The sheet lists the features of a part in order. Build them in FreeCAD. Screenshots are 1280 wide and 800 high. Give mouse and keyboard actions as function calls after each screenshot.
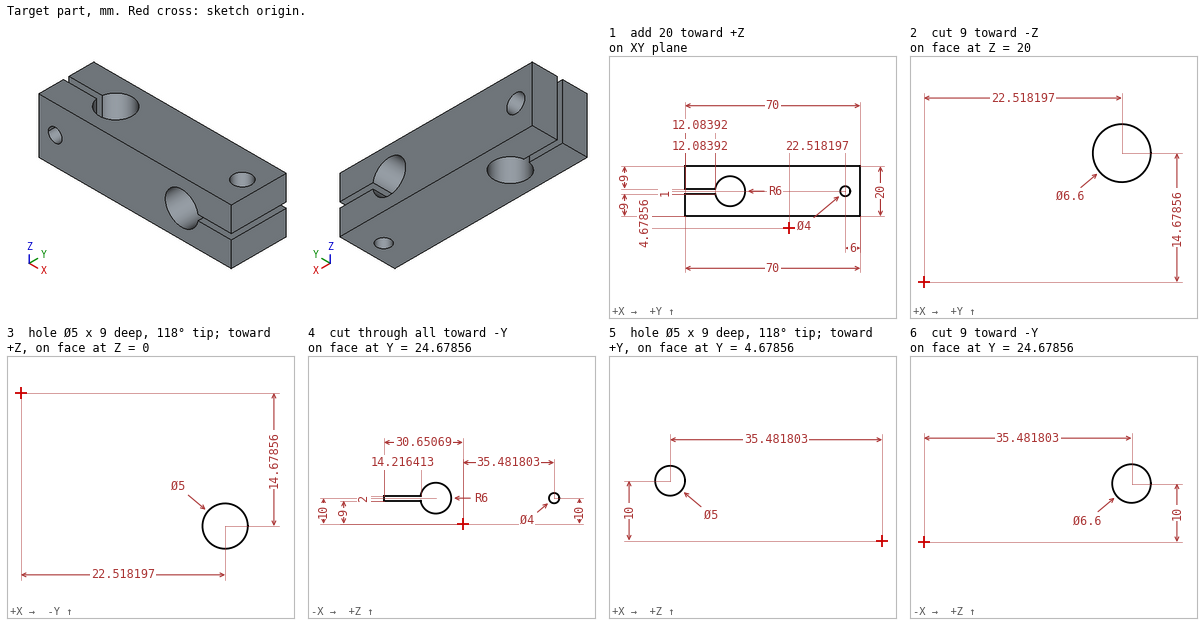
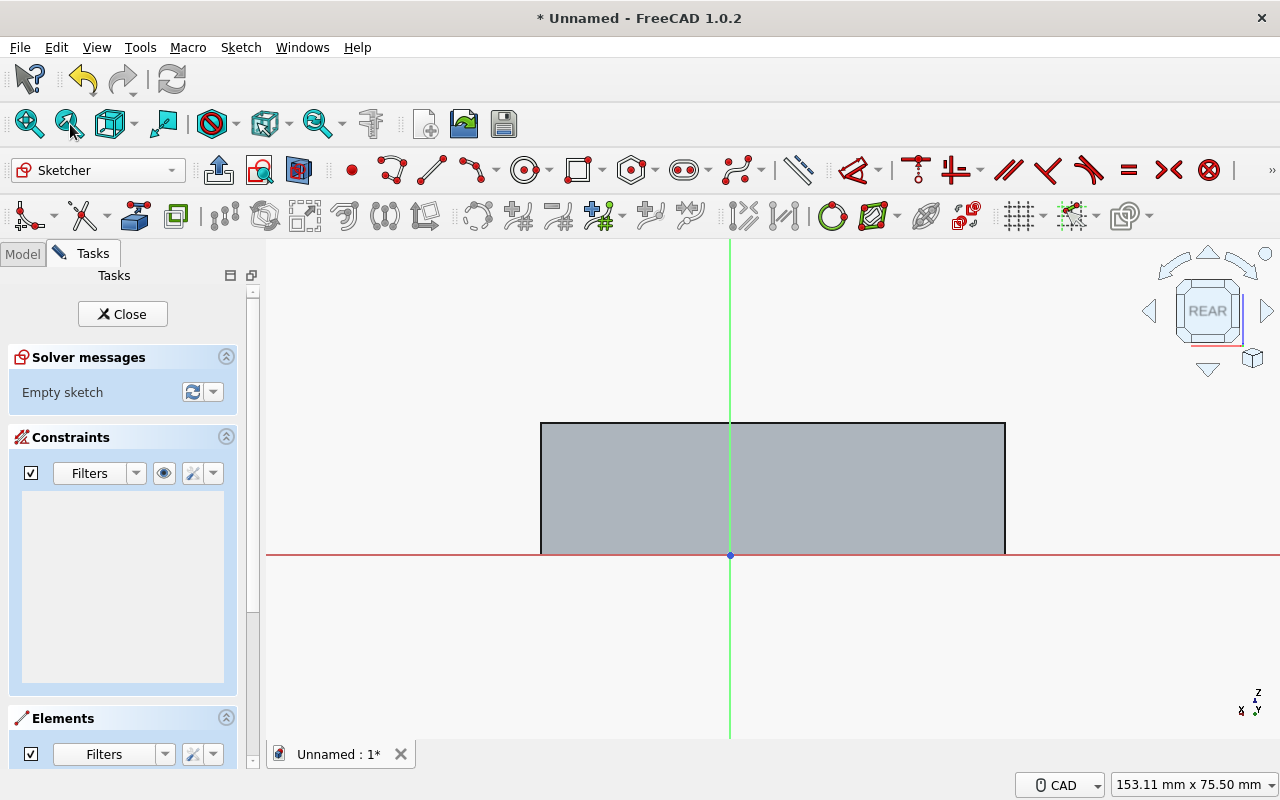
click(392, 170)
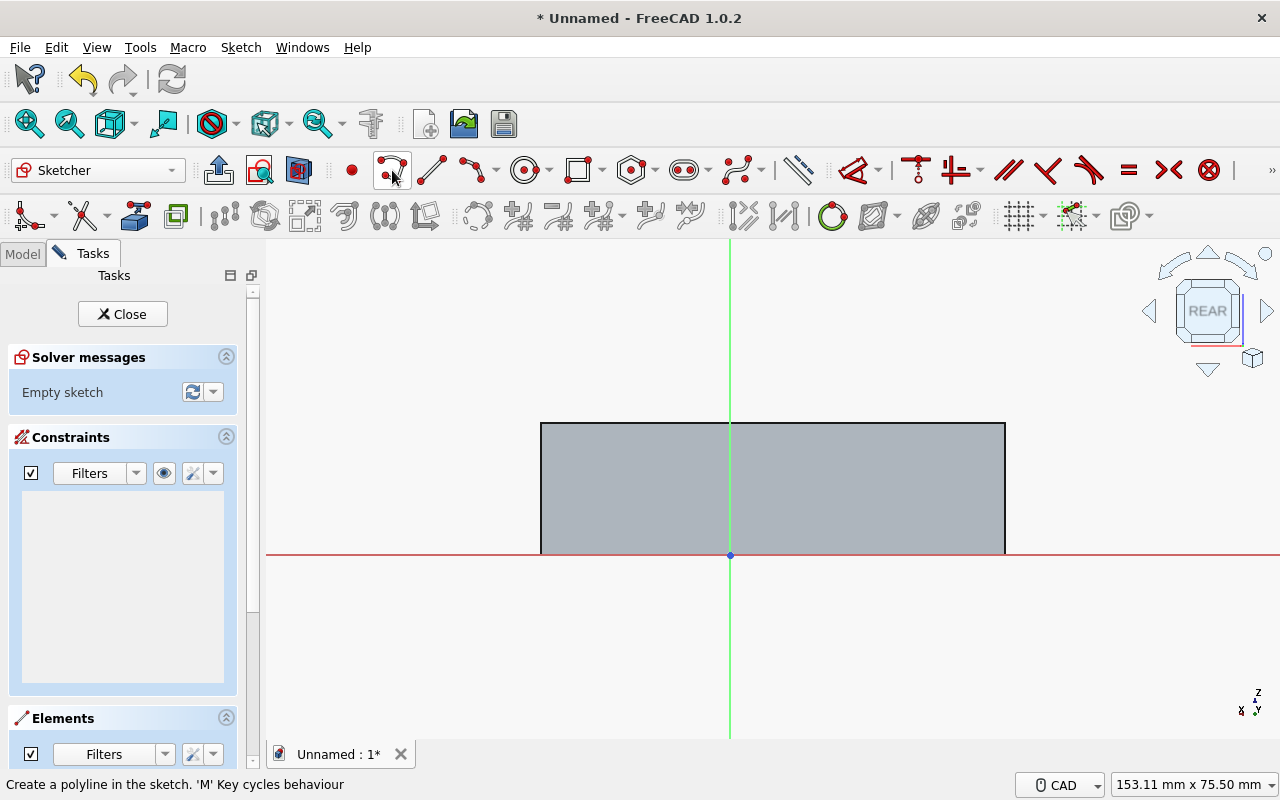
click(621, 482)
click(527, 482)
click(527, 496)
click(621, 496)
right_click(621, 496)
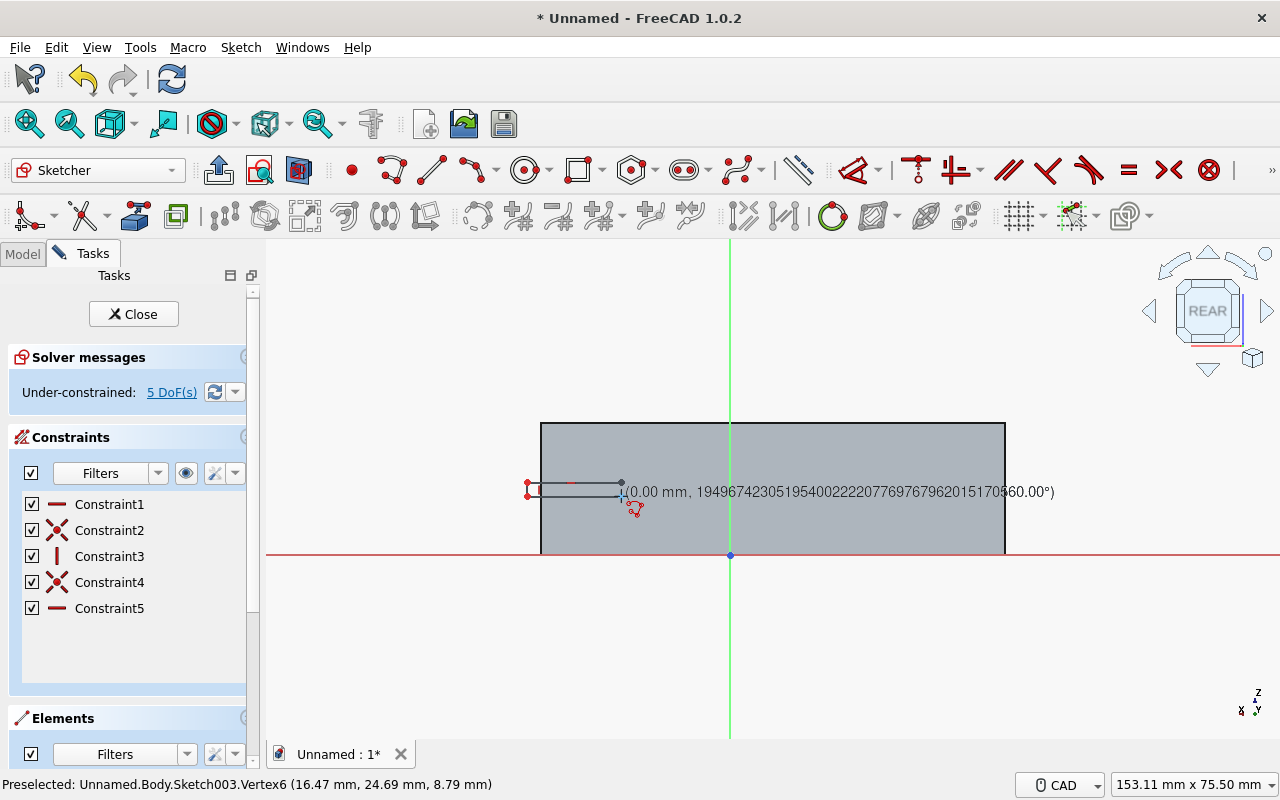
click(472, 170)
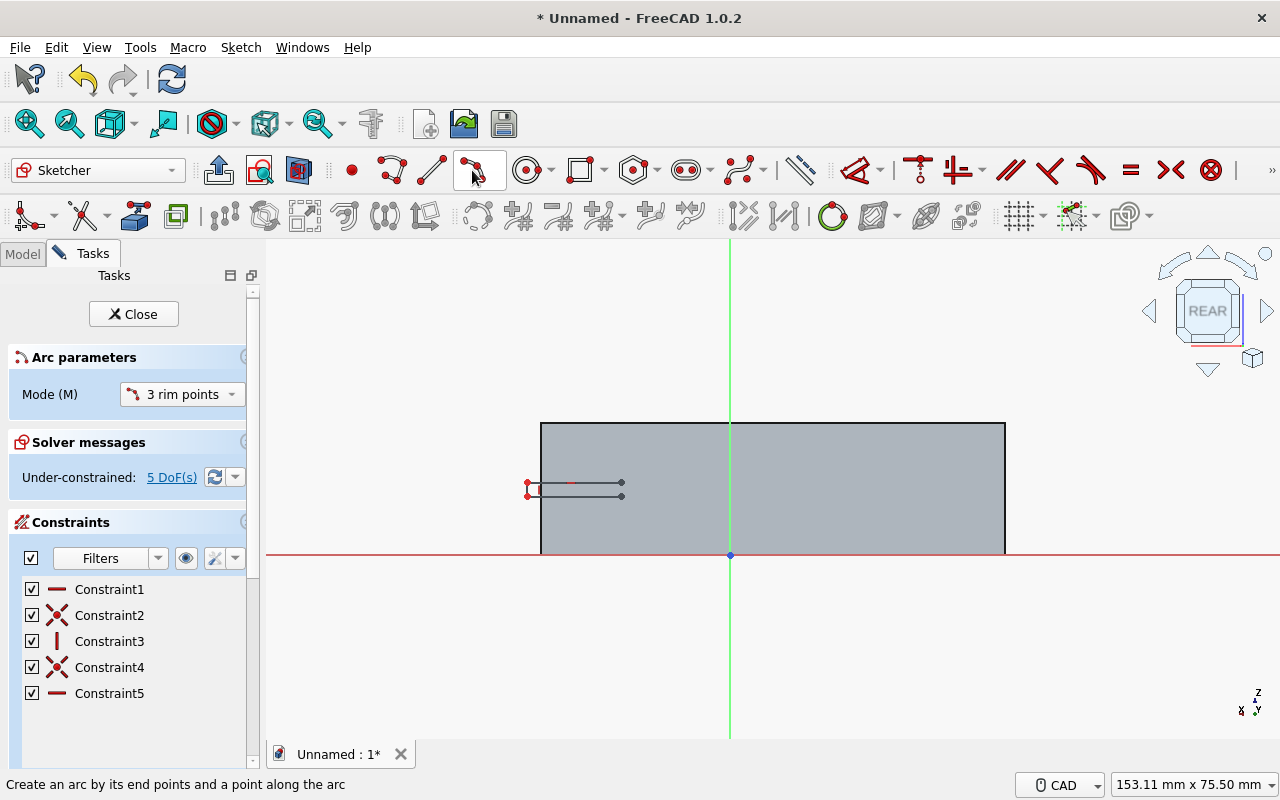
click(621, 497)
click(621, 483)
click(700, 489)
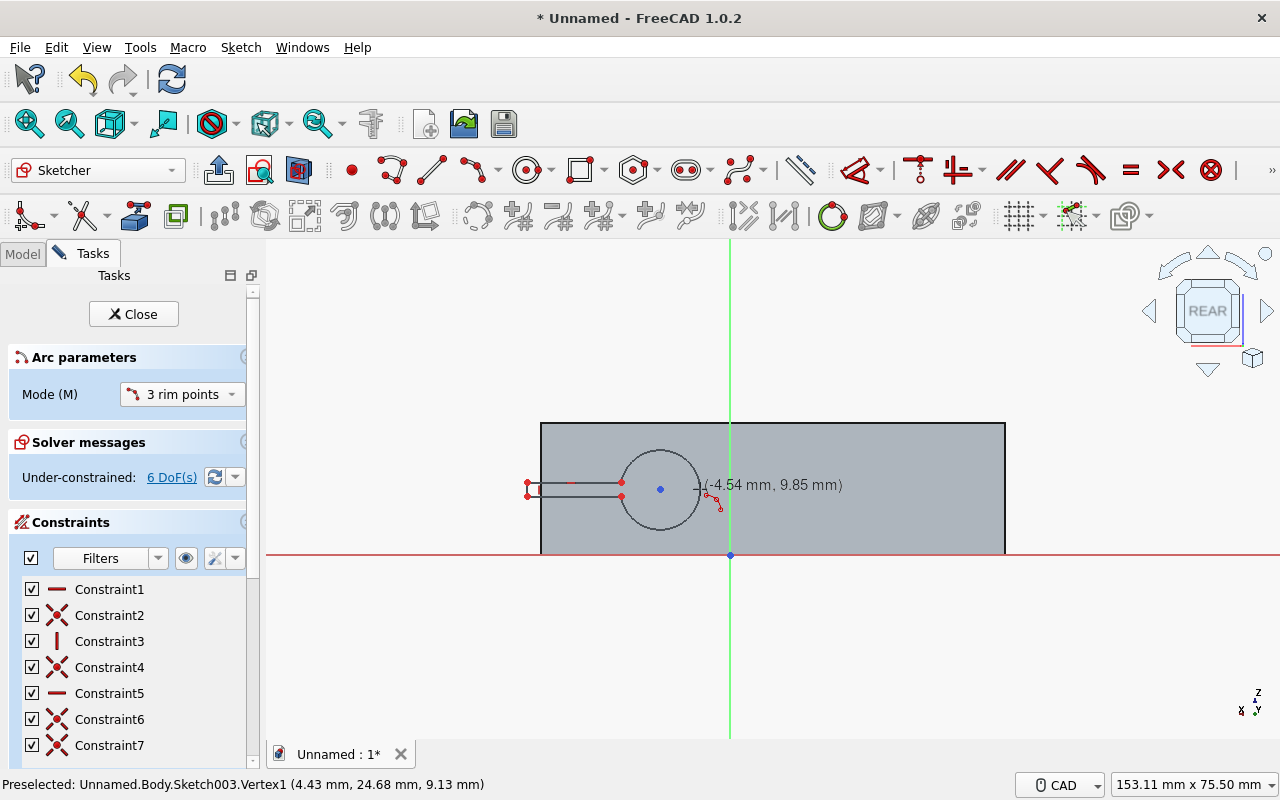
click(528, 170)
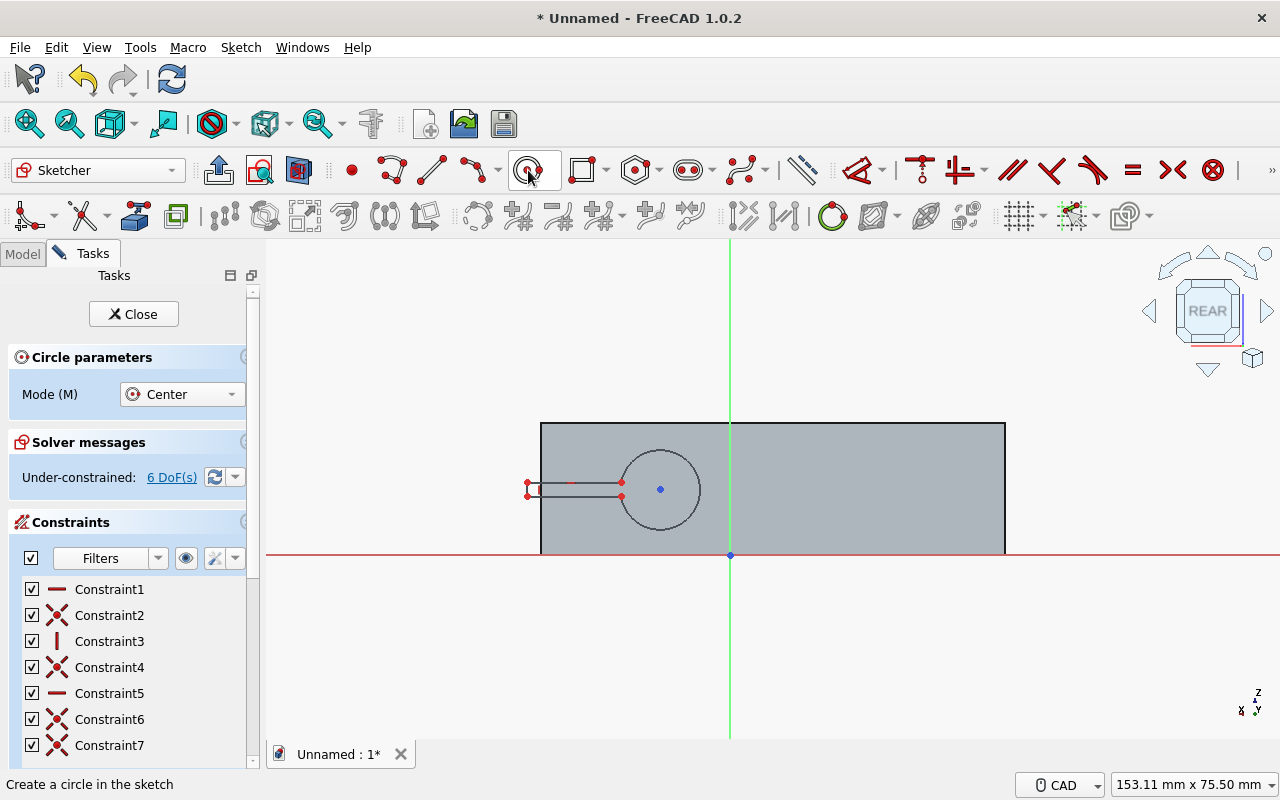
scroll(965, 489, up, 3)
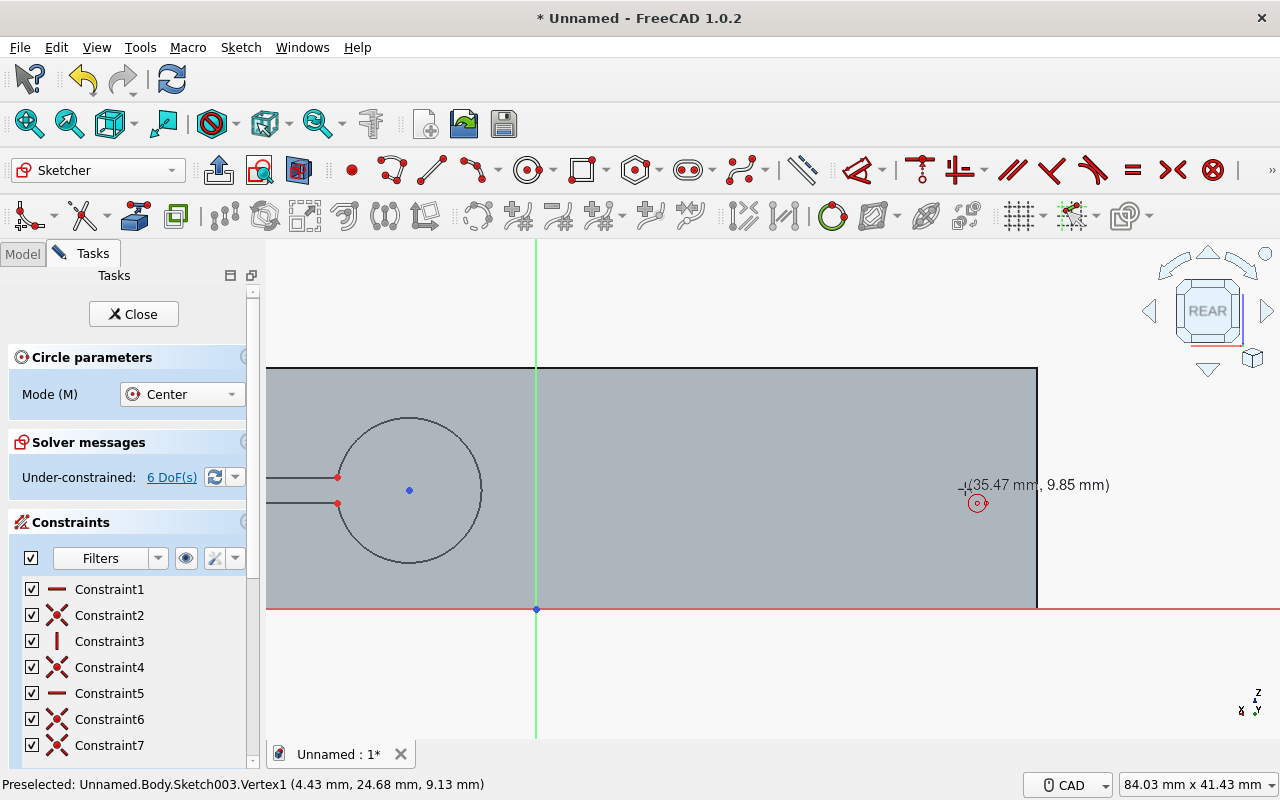
click(965, 489)
click(982, 472)
key(Escape)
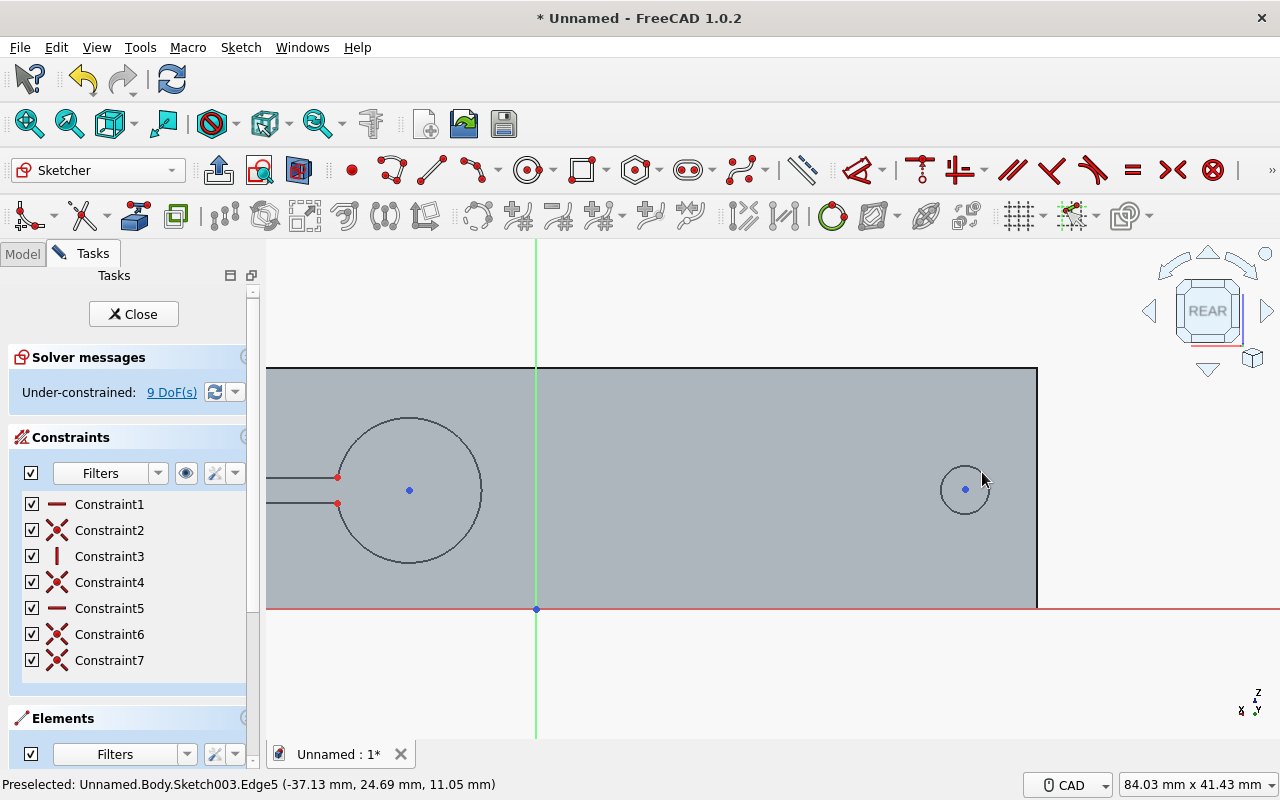
click(858, 170)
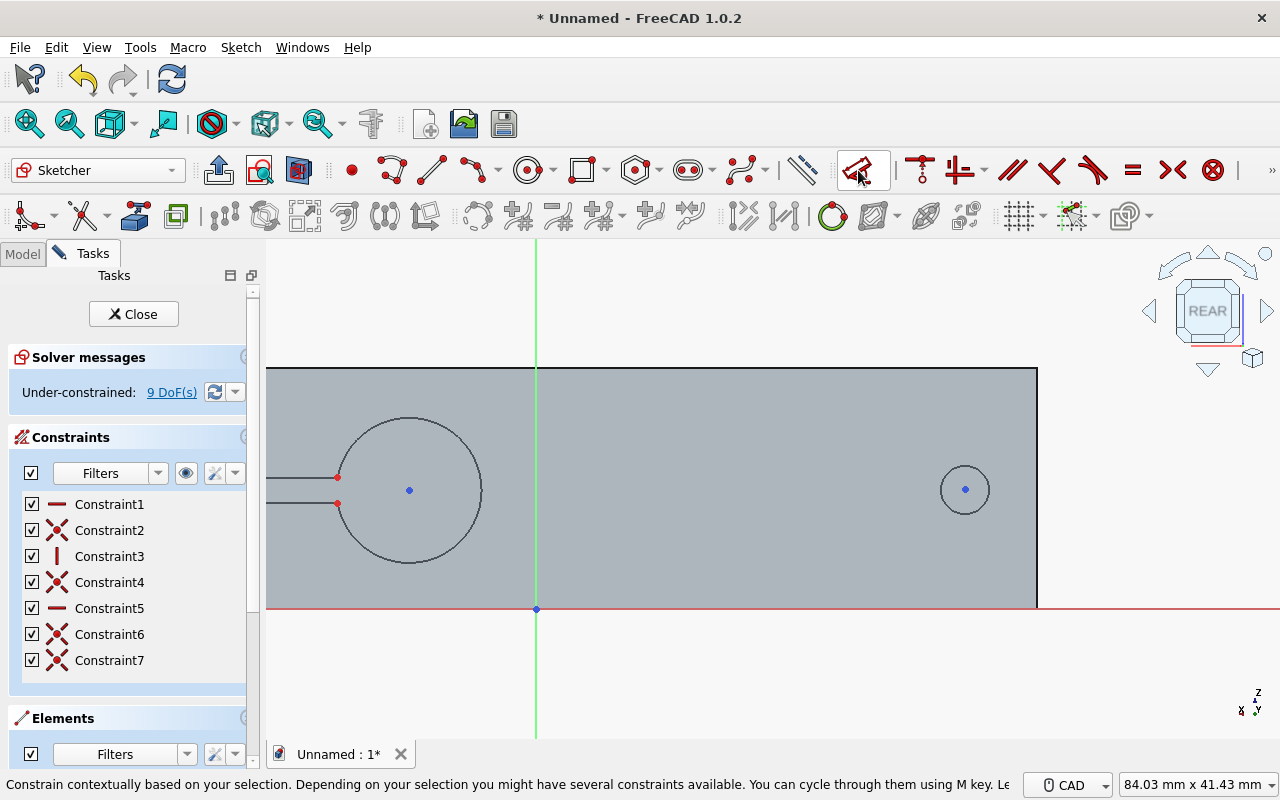
click(436, 558)
click(448, 588)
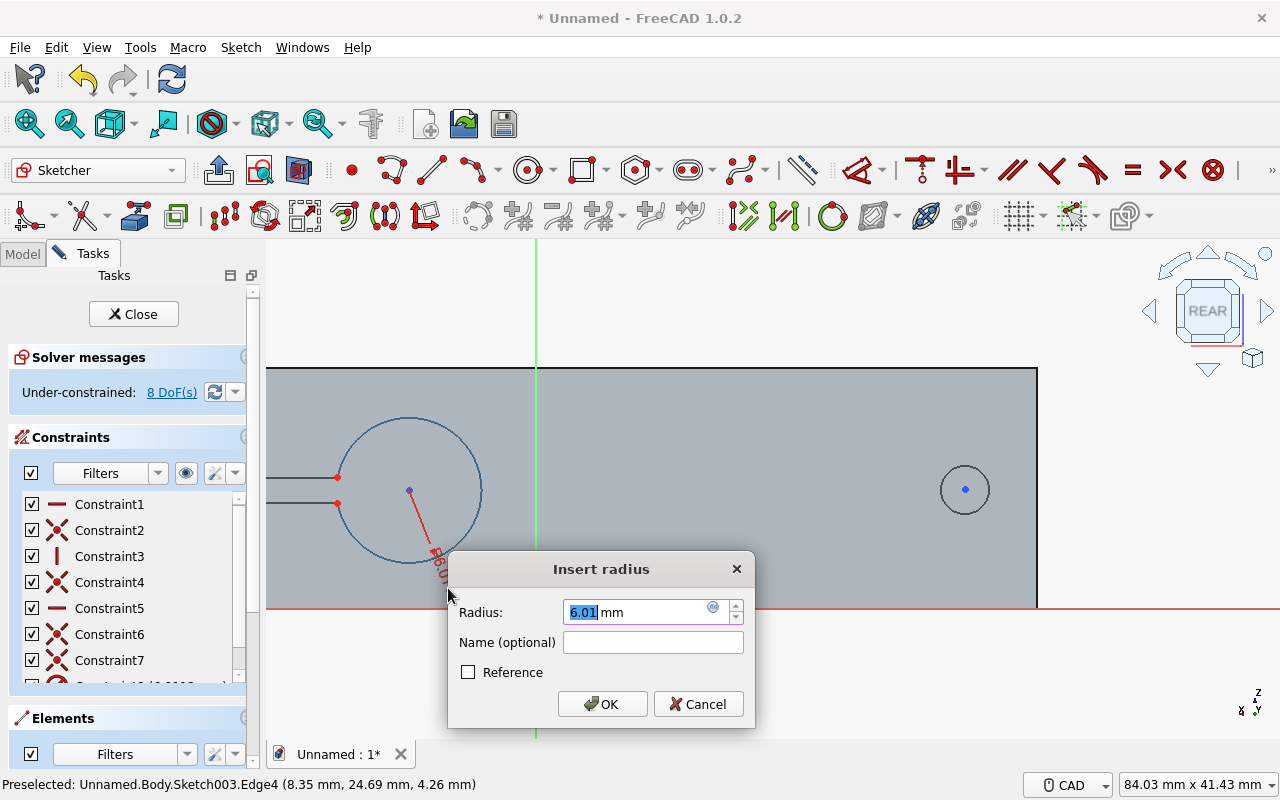
text(6)
key(Return)